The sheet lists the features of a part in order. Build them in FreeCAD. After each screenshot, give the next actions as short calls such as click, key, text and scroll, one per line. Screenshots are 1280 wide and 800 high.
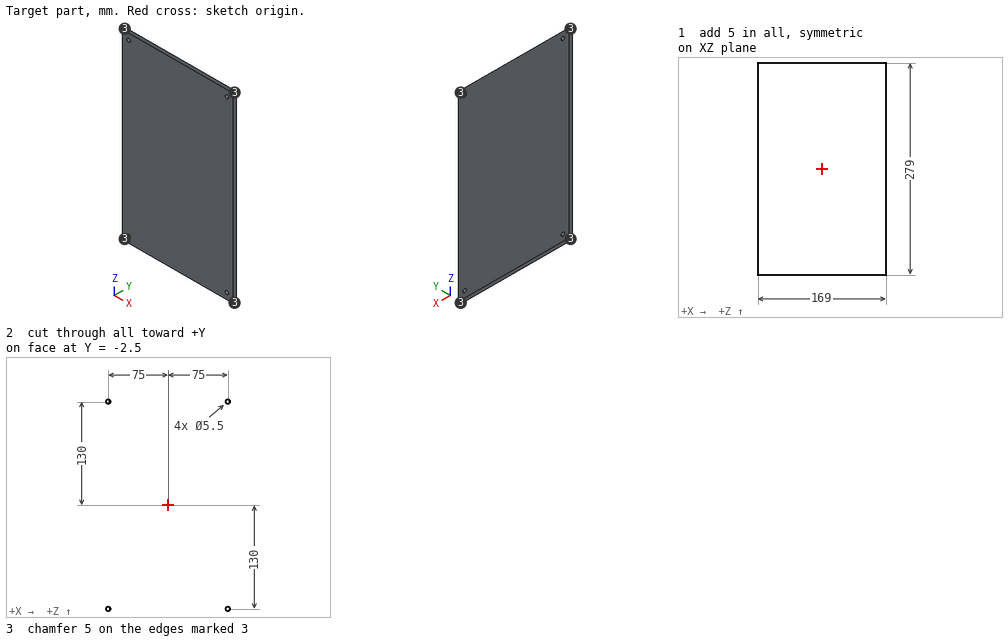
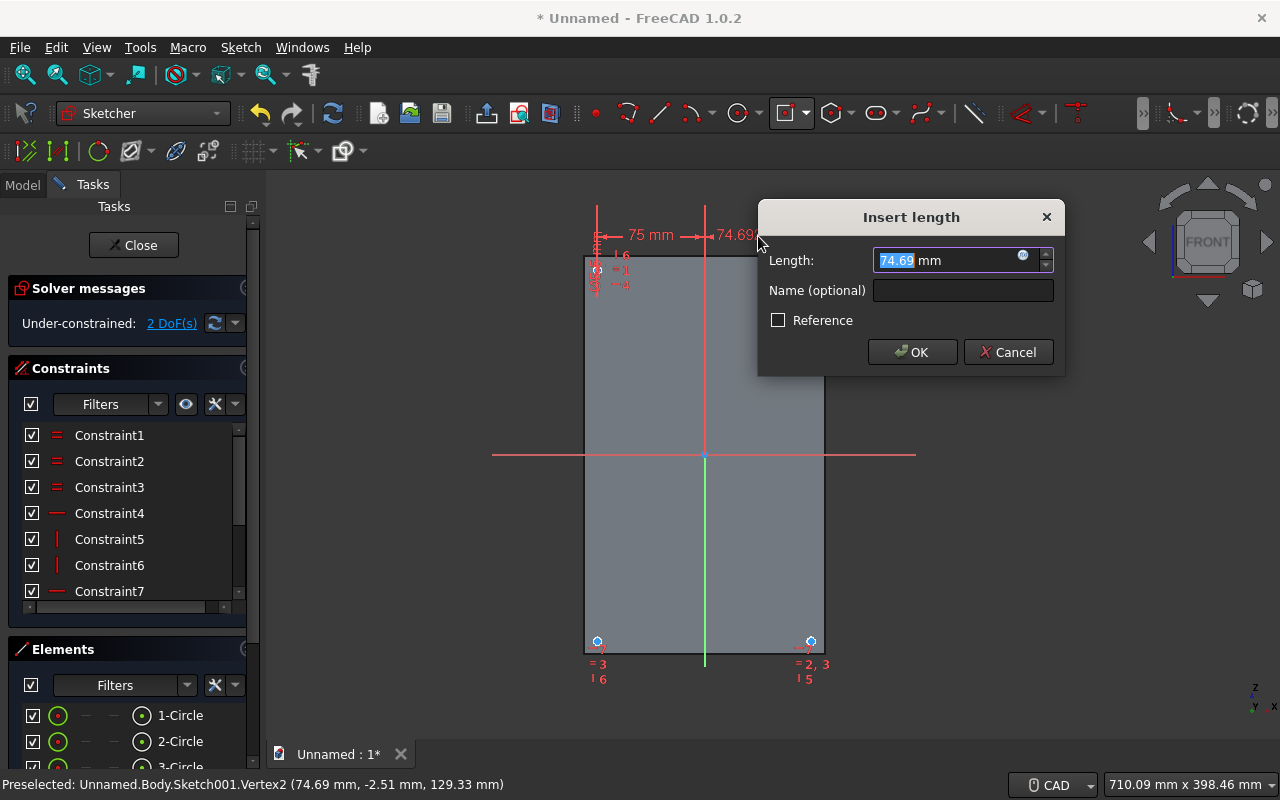
text(75)
key(Return)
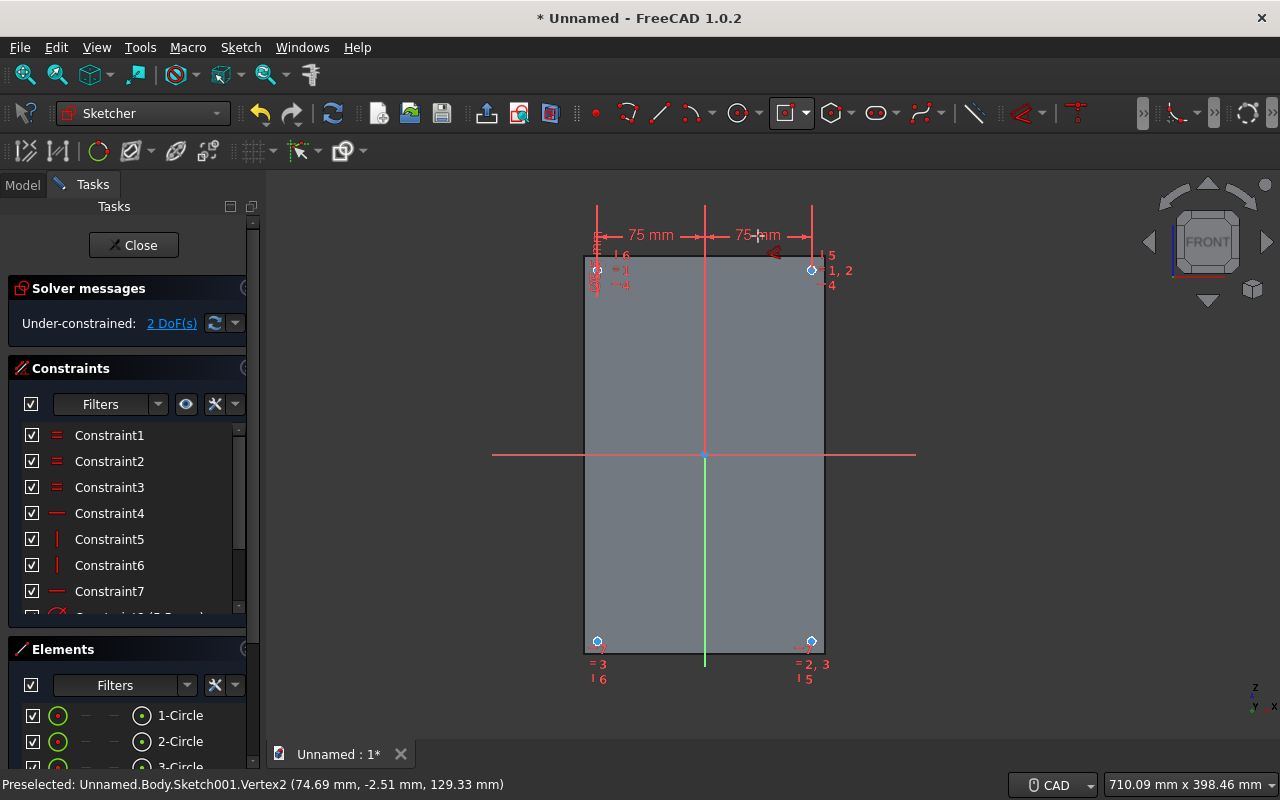
click(597, 270)
click(563, 363)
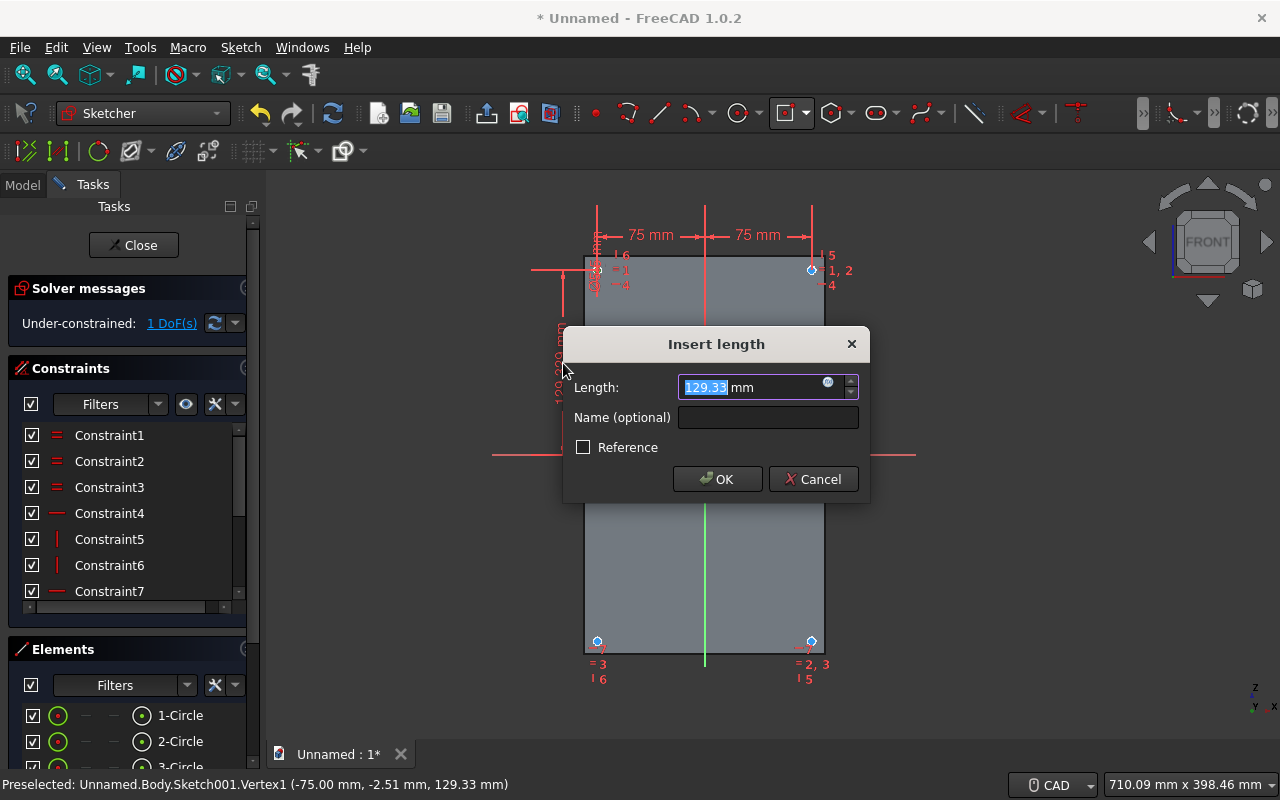
text(130)
key(Return)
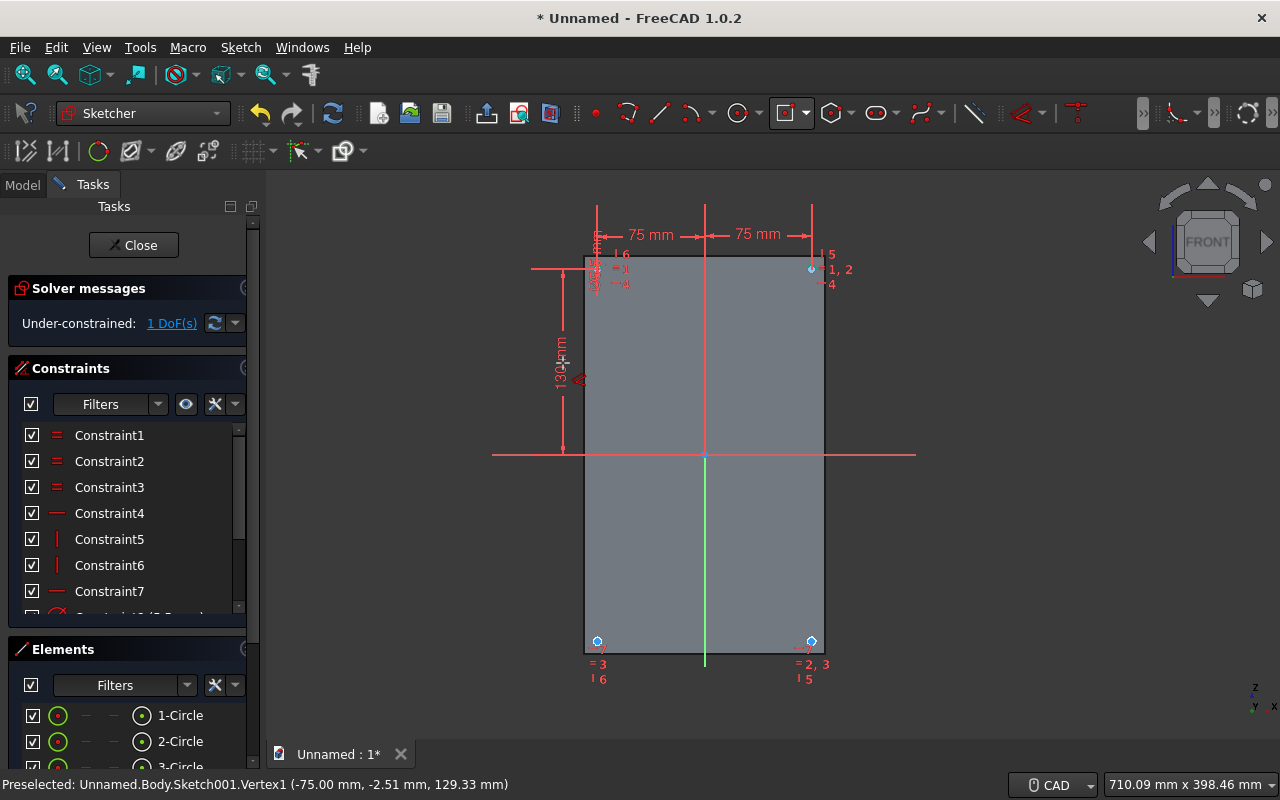
click(812, 641)
click(846, 548)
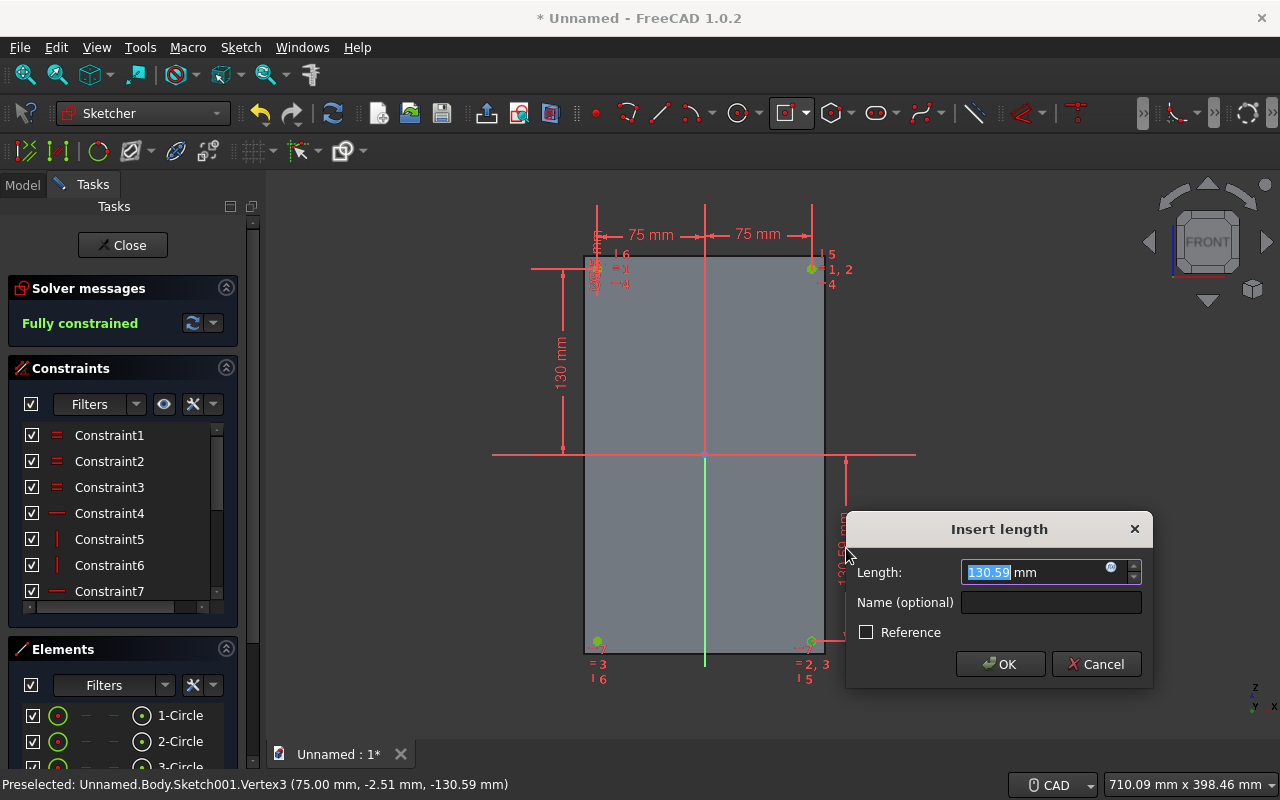
text(130)
key(Return)
key(Escape)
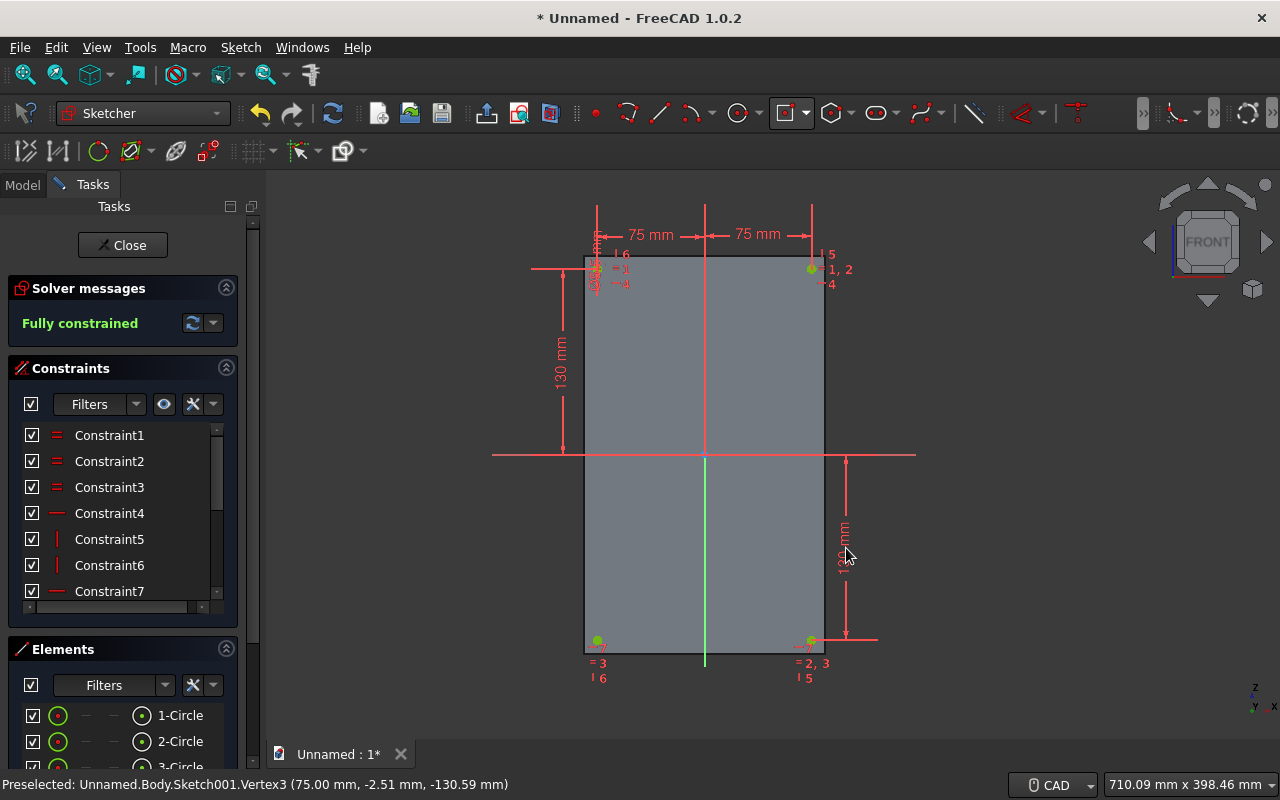
click(123, 245)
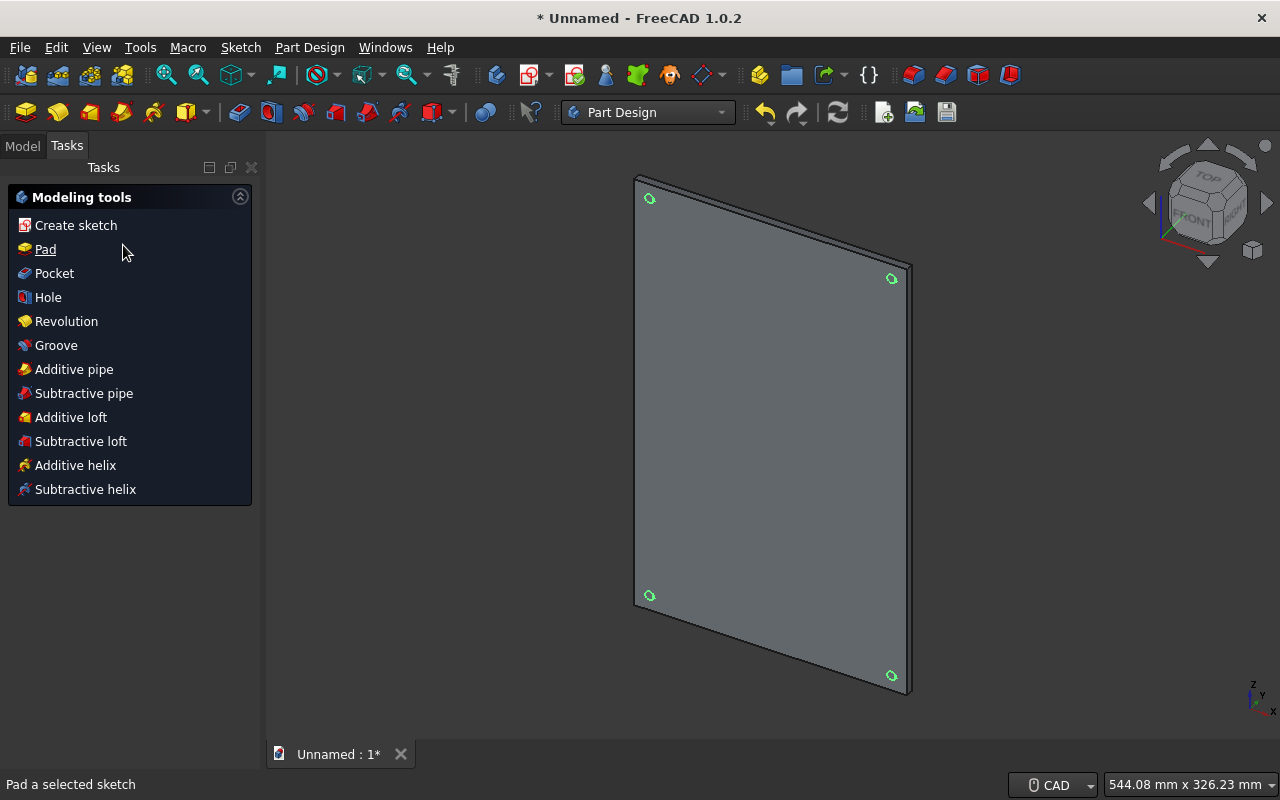
click(240, 112)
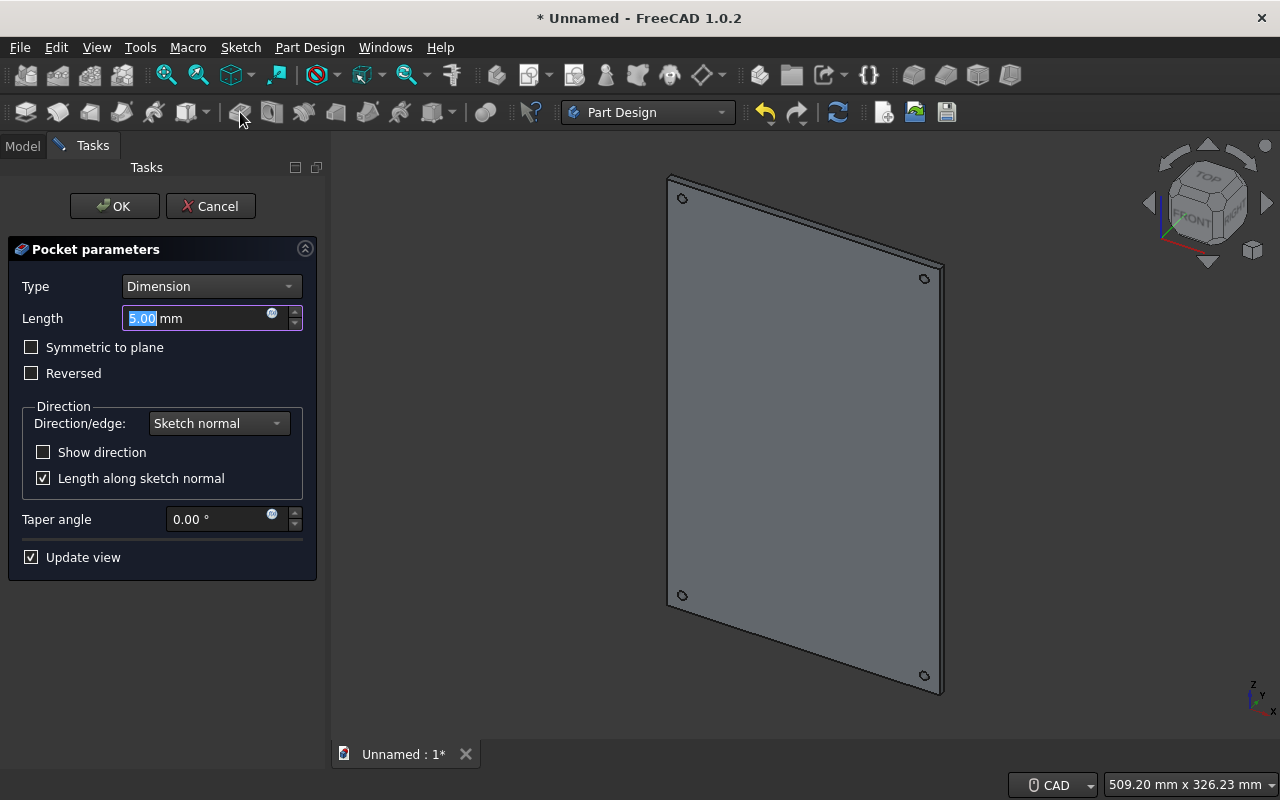
click(212, 286)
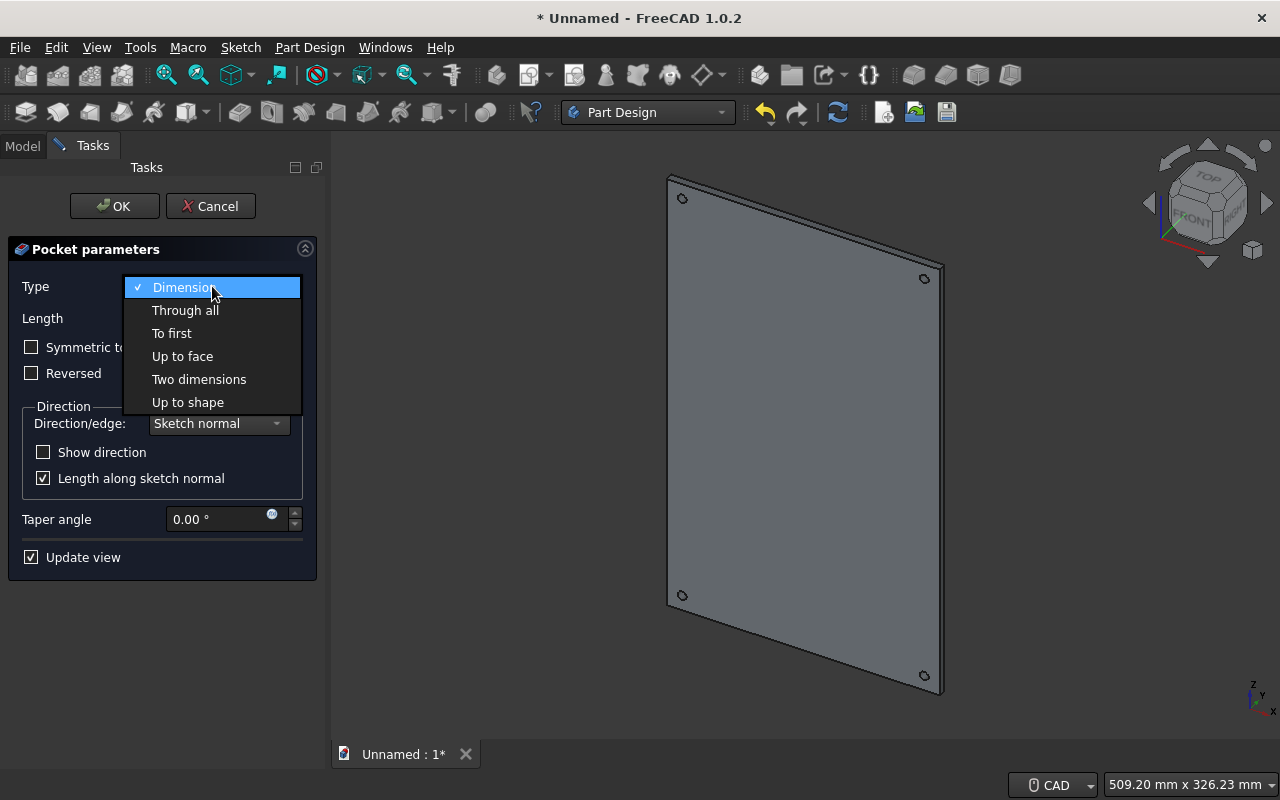
click(212, 310)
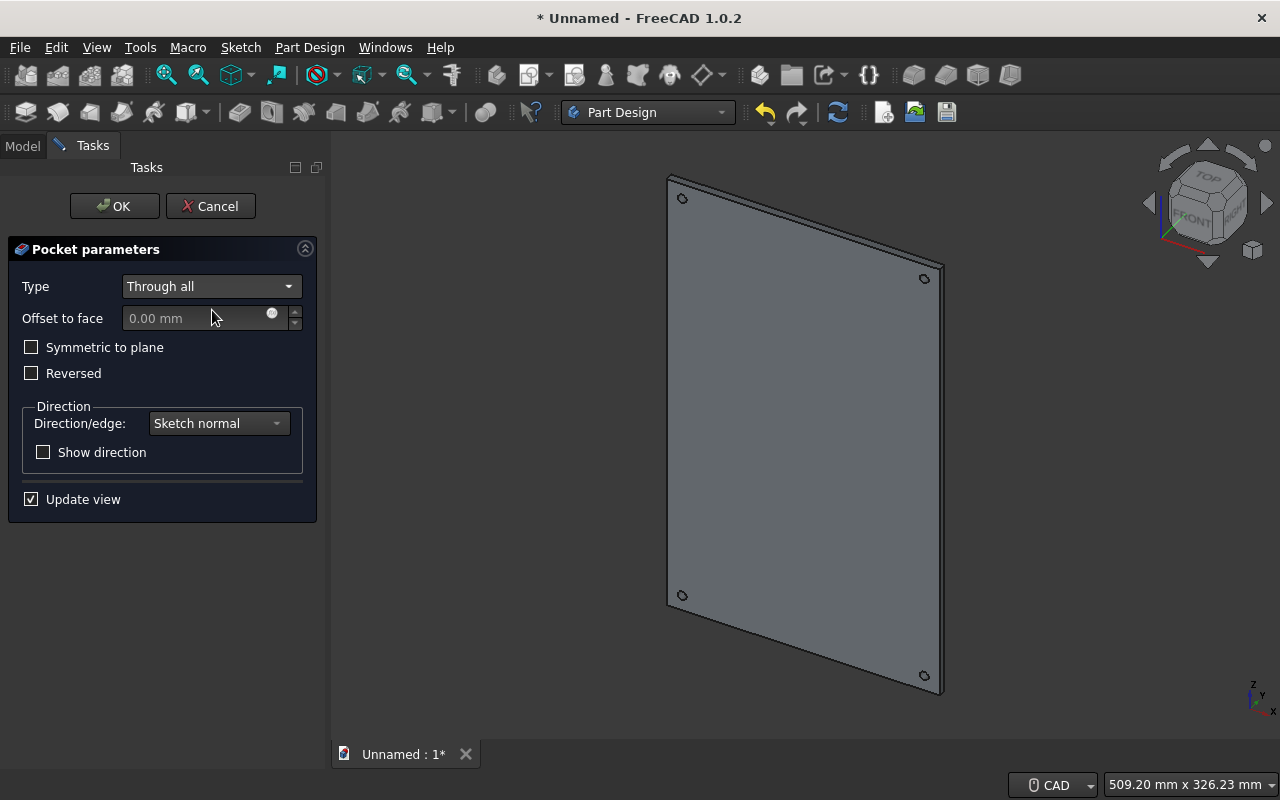
click(115, 206)